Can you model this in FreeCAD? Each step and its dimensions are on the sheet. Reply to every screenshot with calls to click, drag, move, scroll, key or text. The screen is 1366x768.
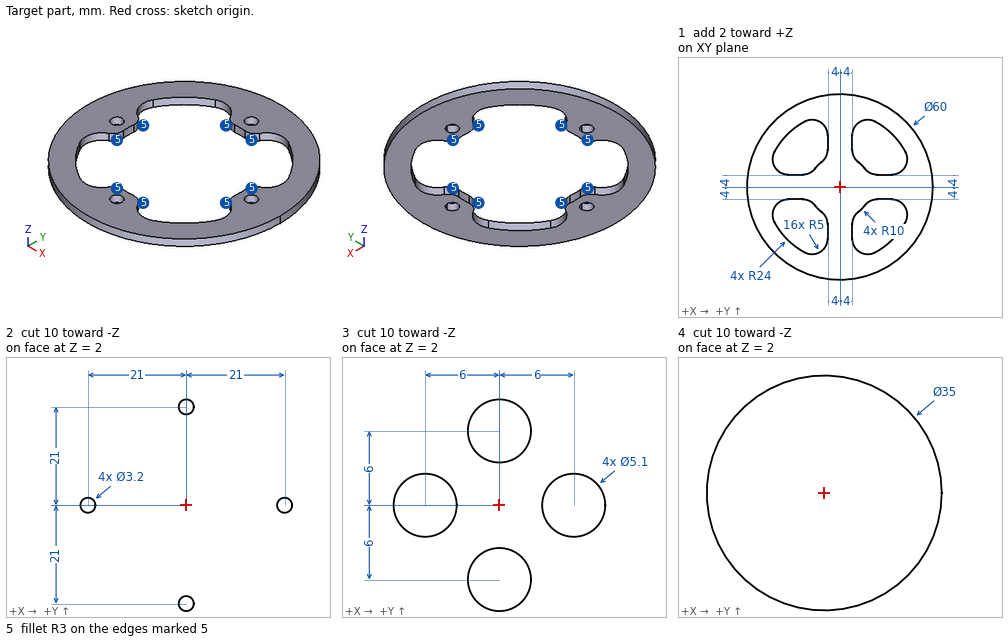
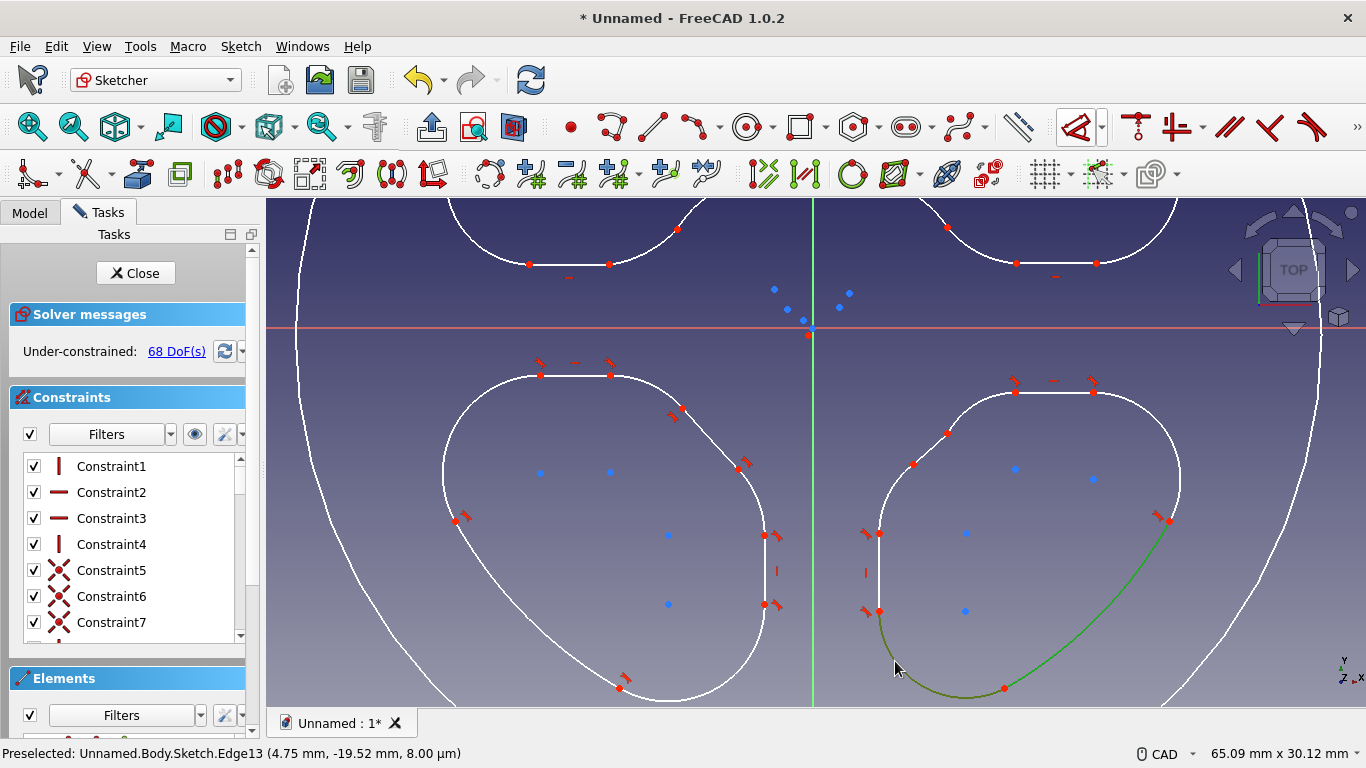
key(t)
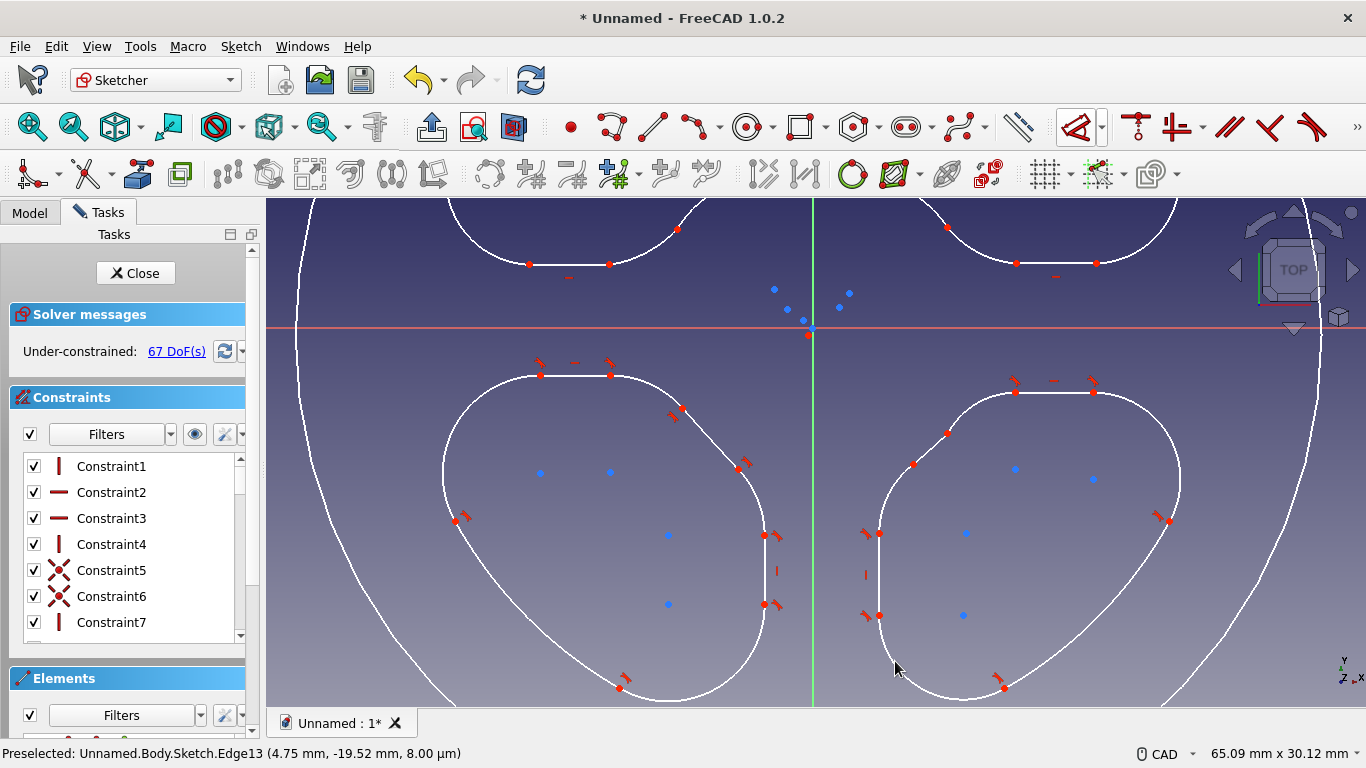
click(897, 481)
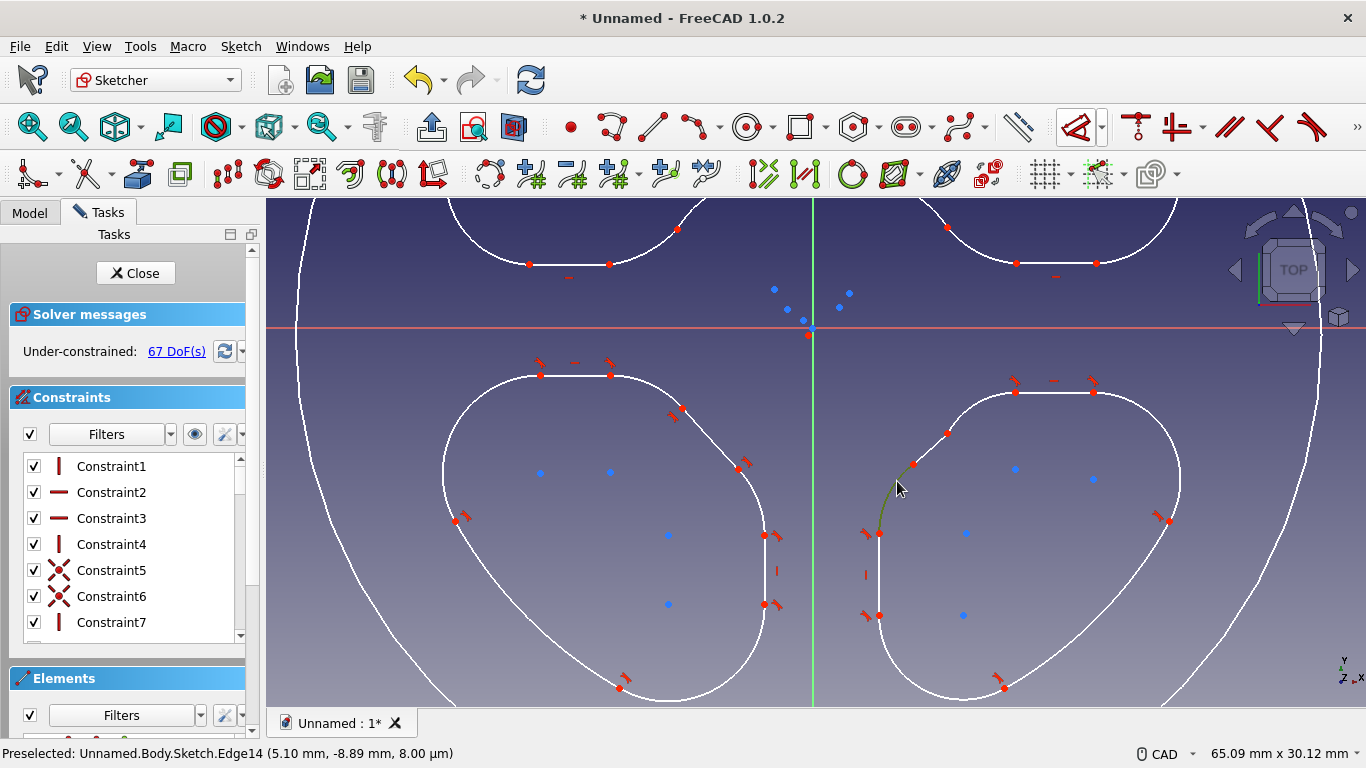
click(924, 455)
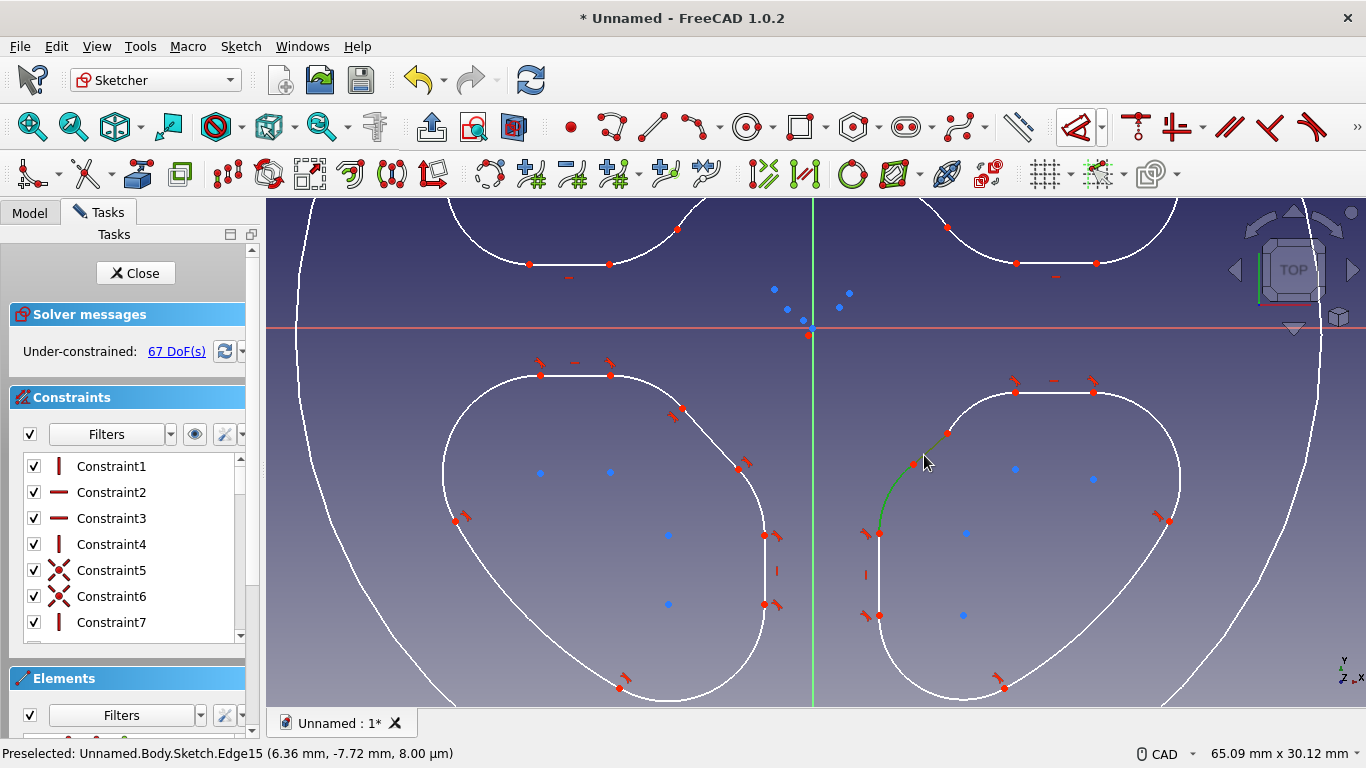
click(1312, 128)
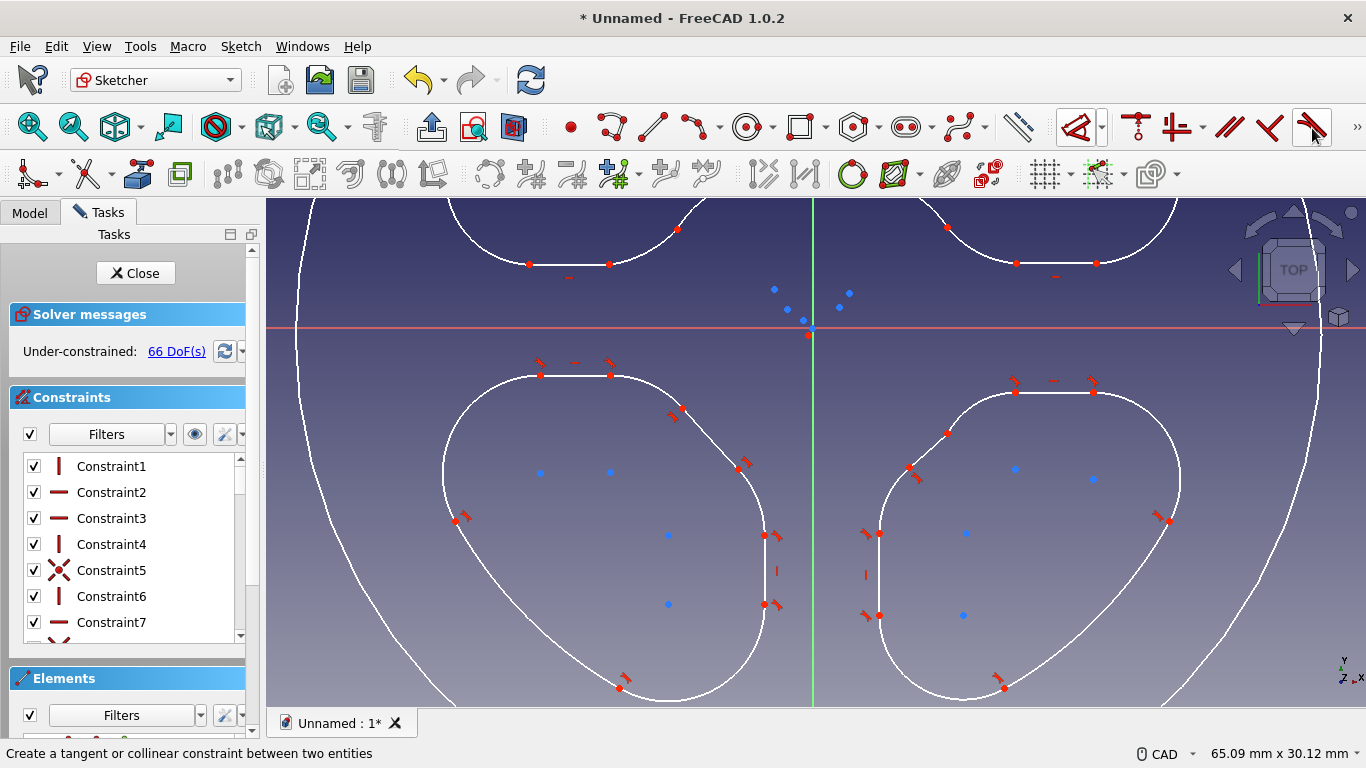
click(921, 458)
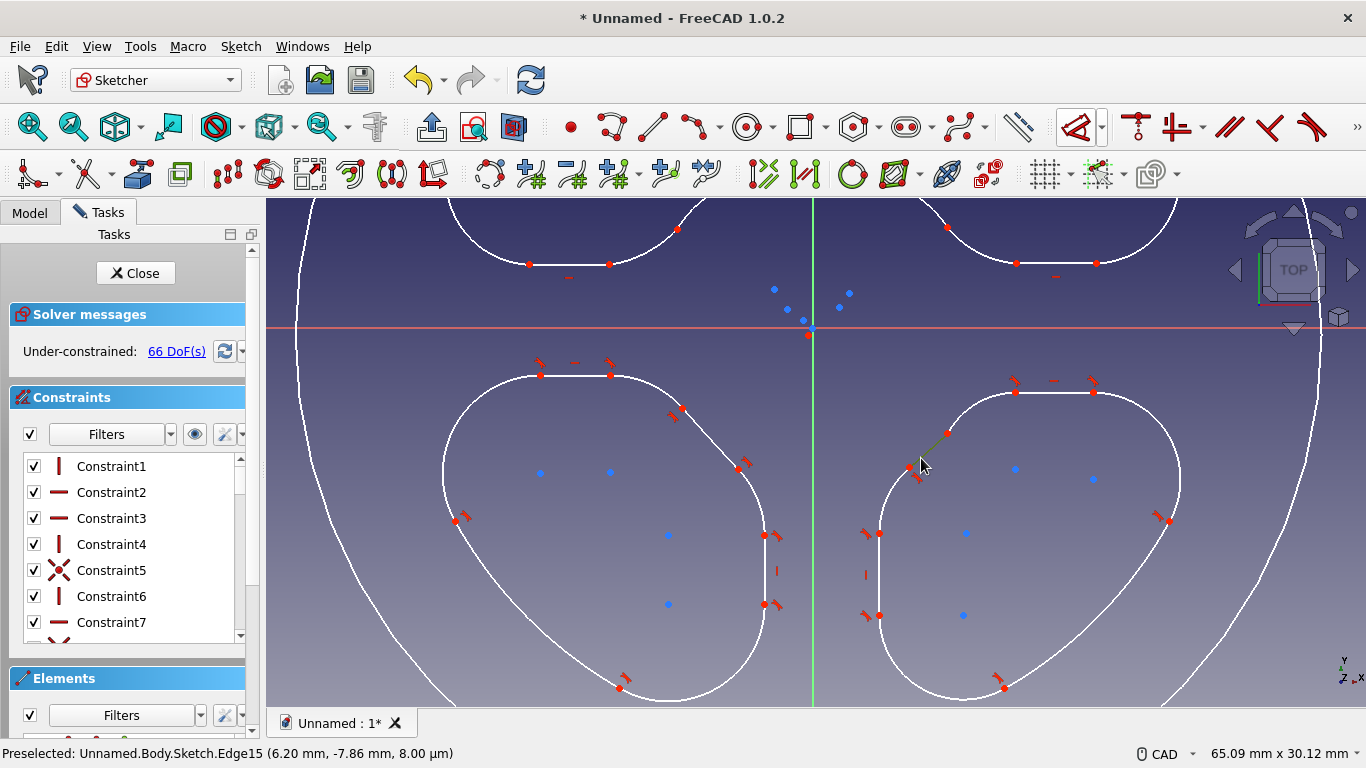
click(991, 397)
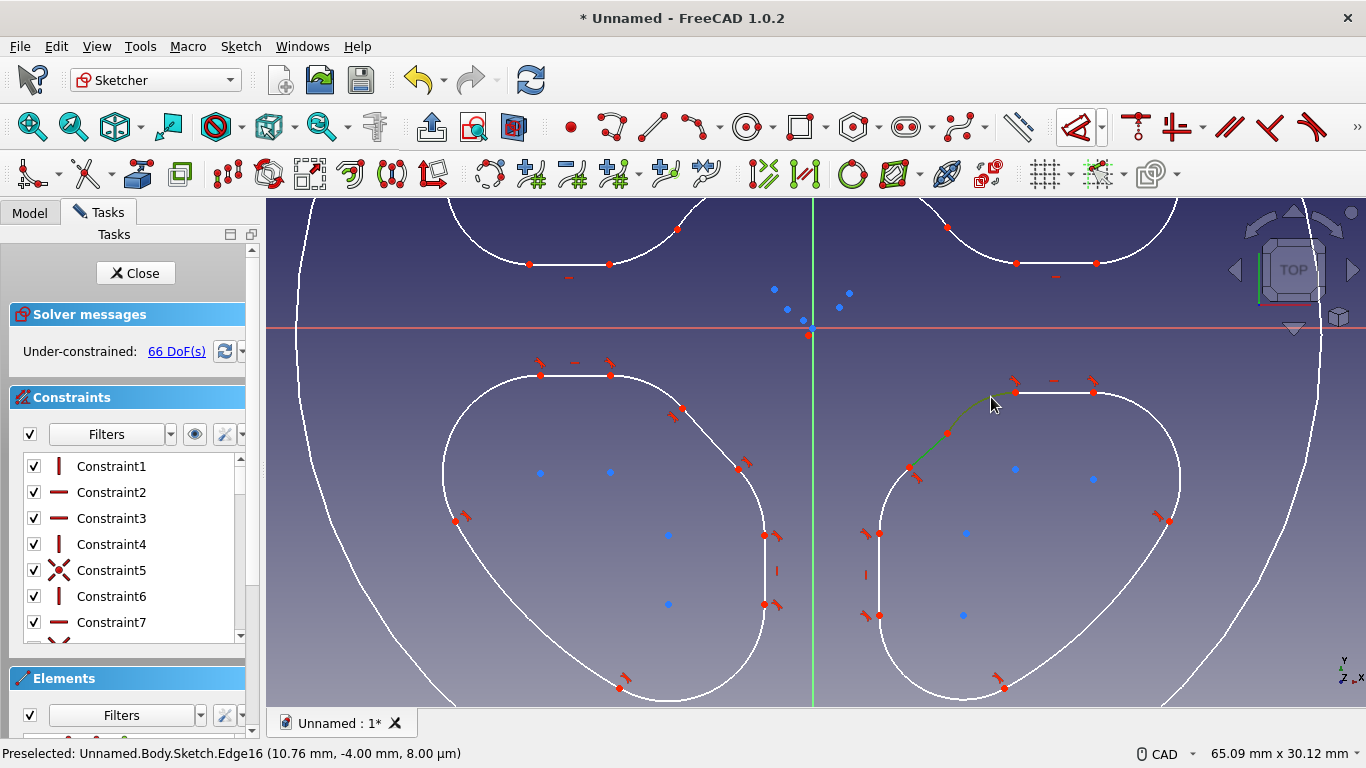
key(t)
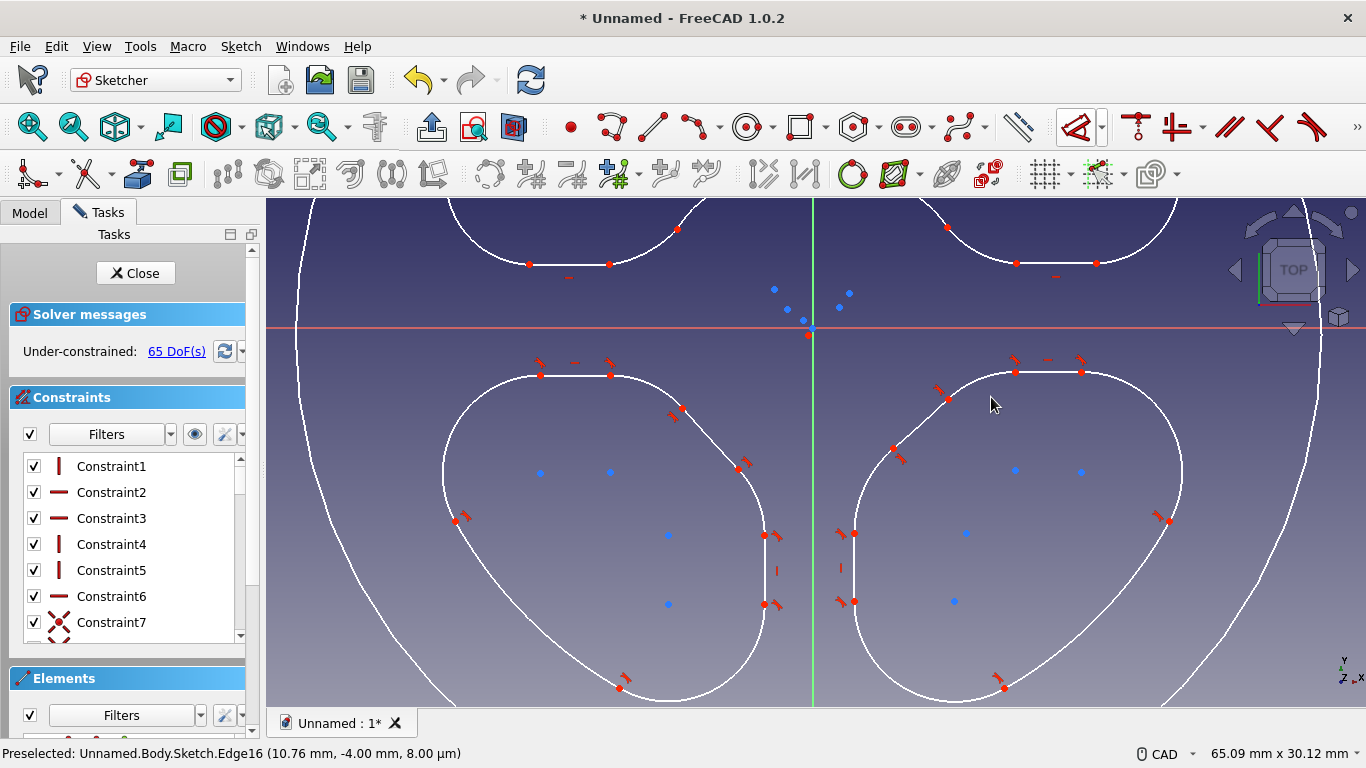
scroll(719, 506, down, 6)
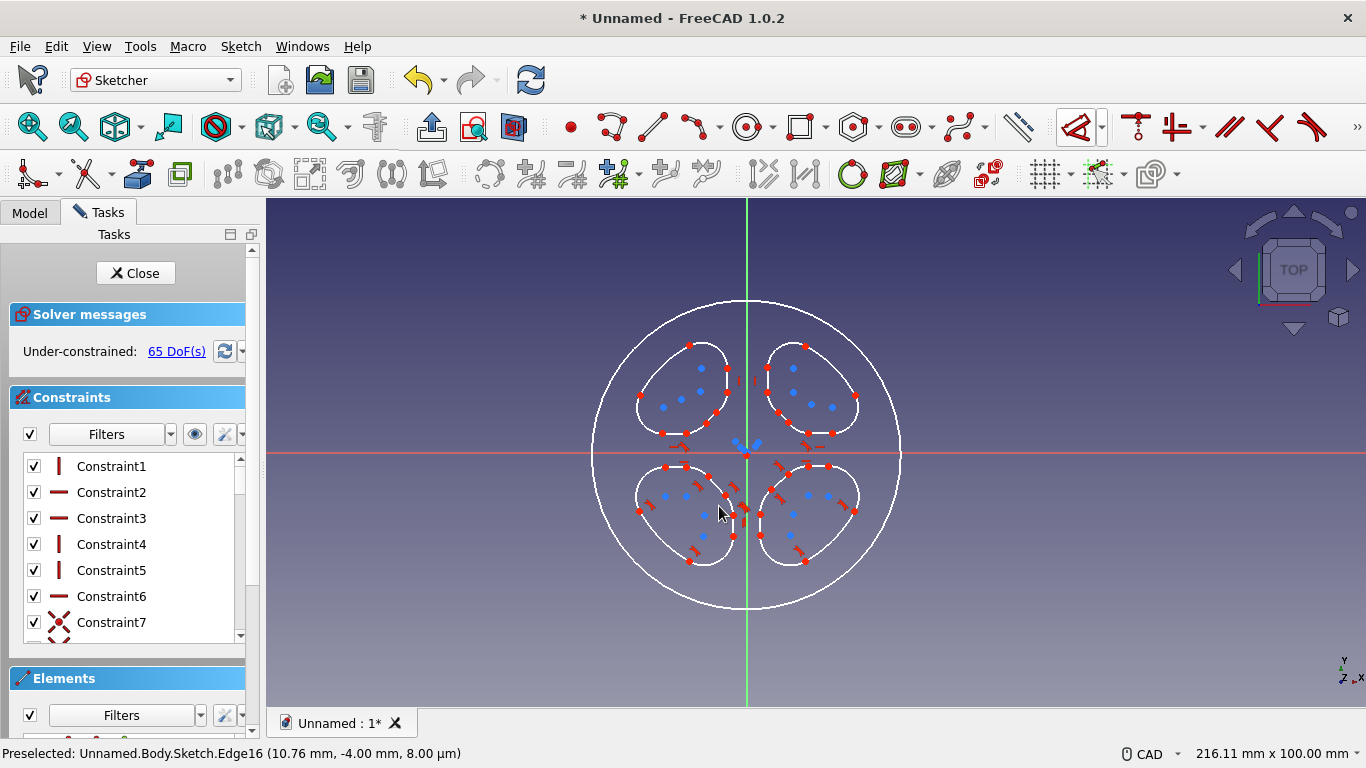
scroll(727, 376, up, 4)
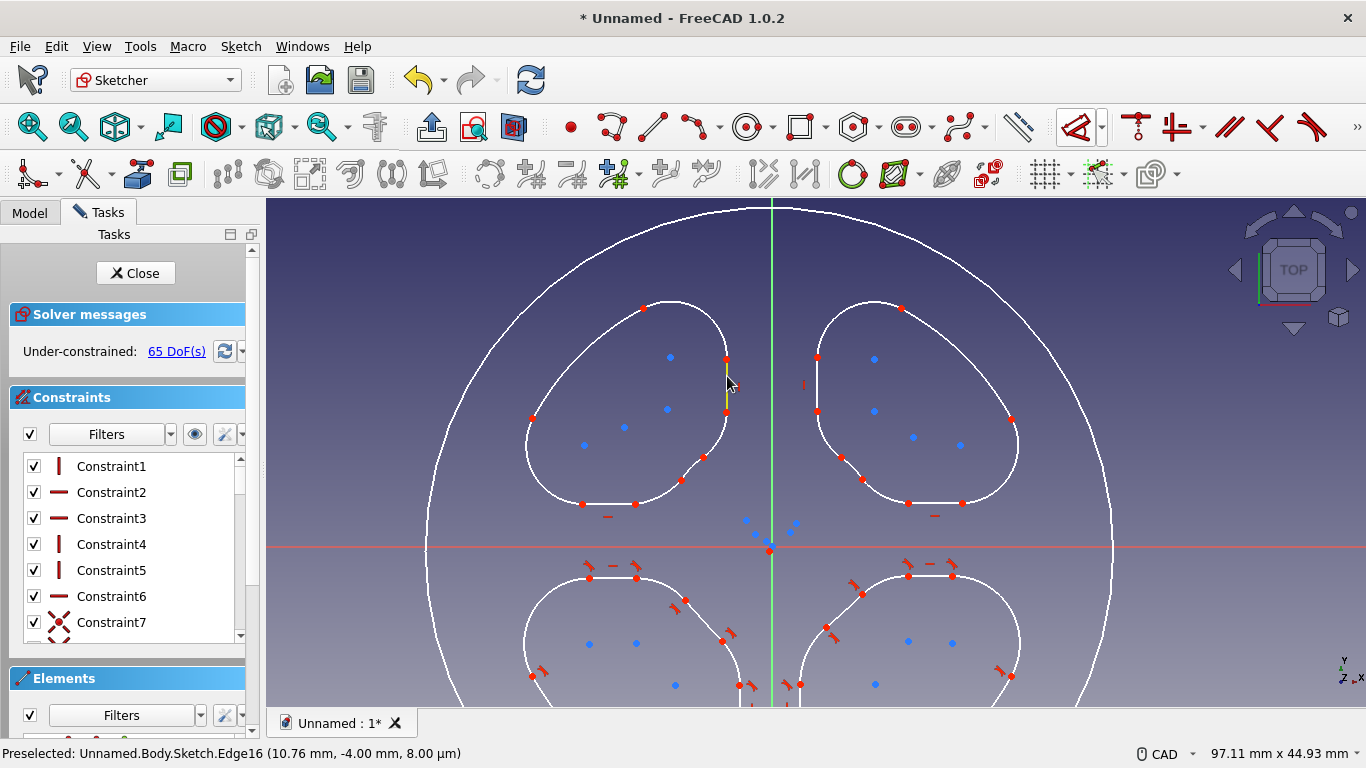
click(727, 375)